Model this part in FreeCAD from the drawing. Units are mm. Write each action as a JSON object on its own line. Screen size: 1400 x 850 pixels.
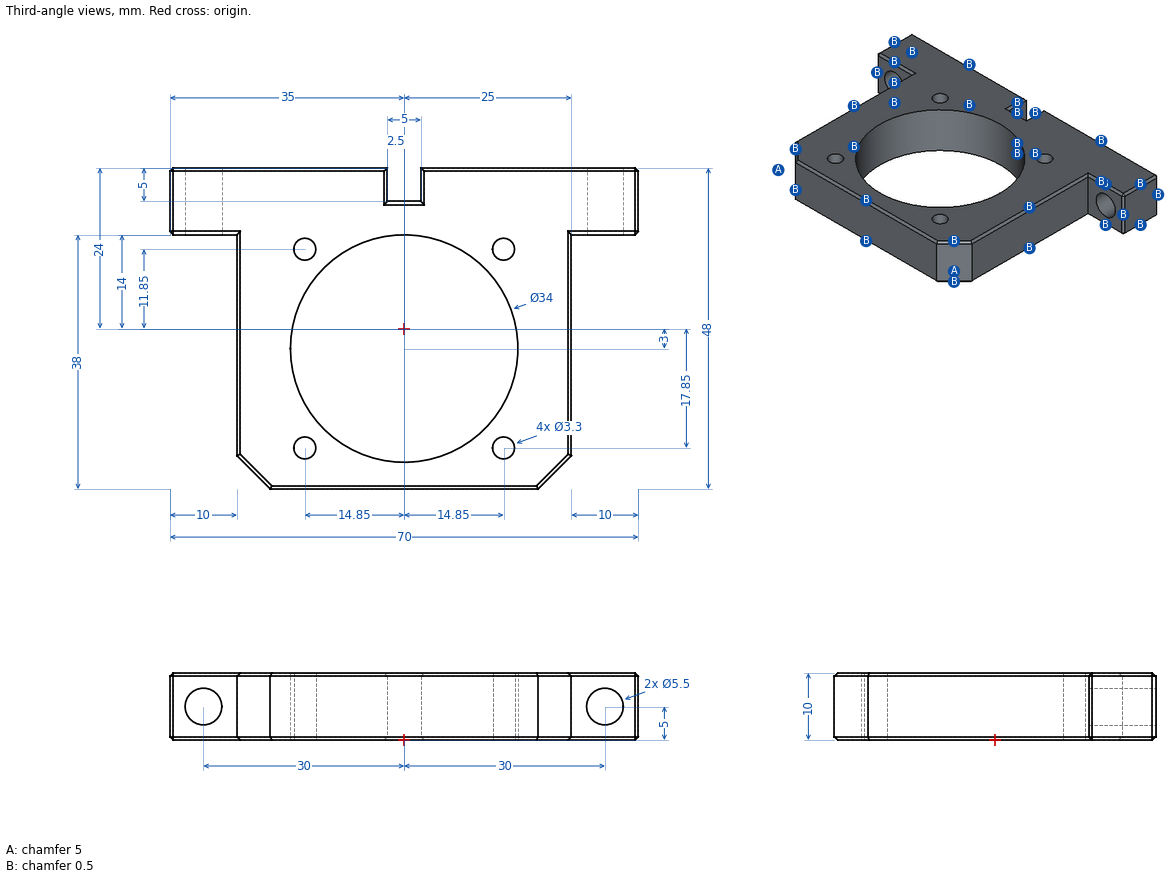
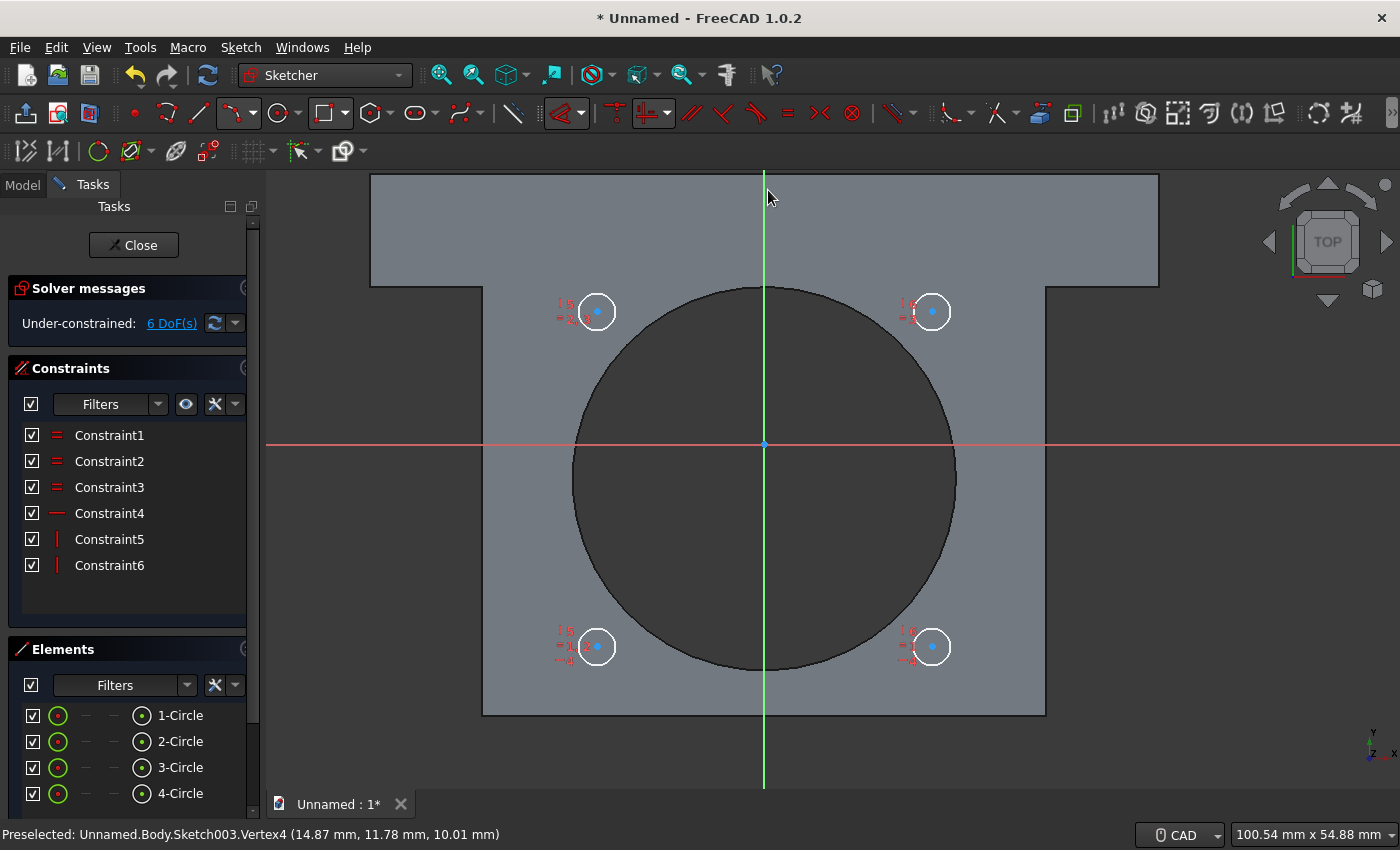
{"action": "left_click", "coordinate": [597, 312]}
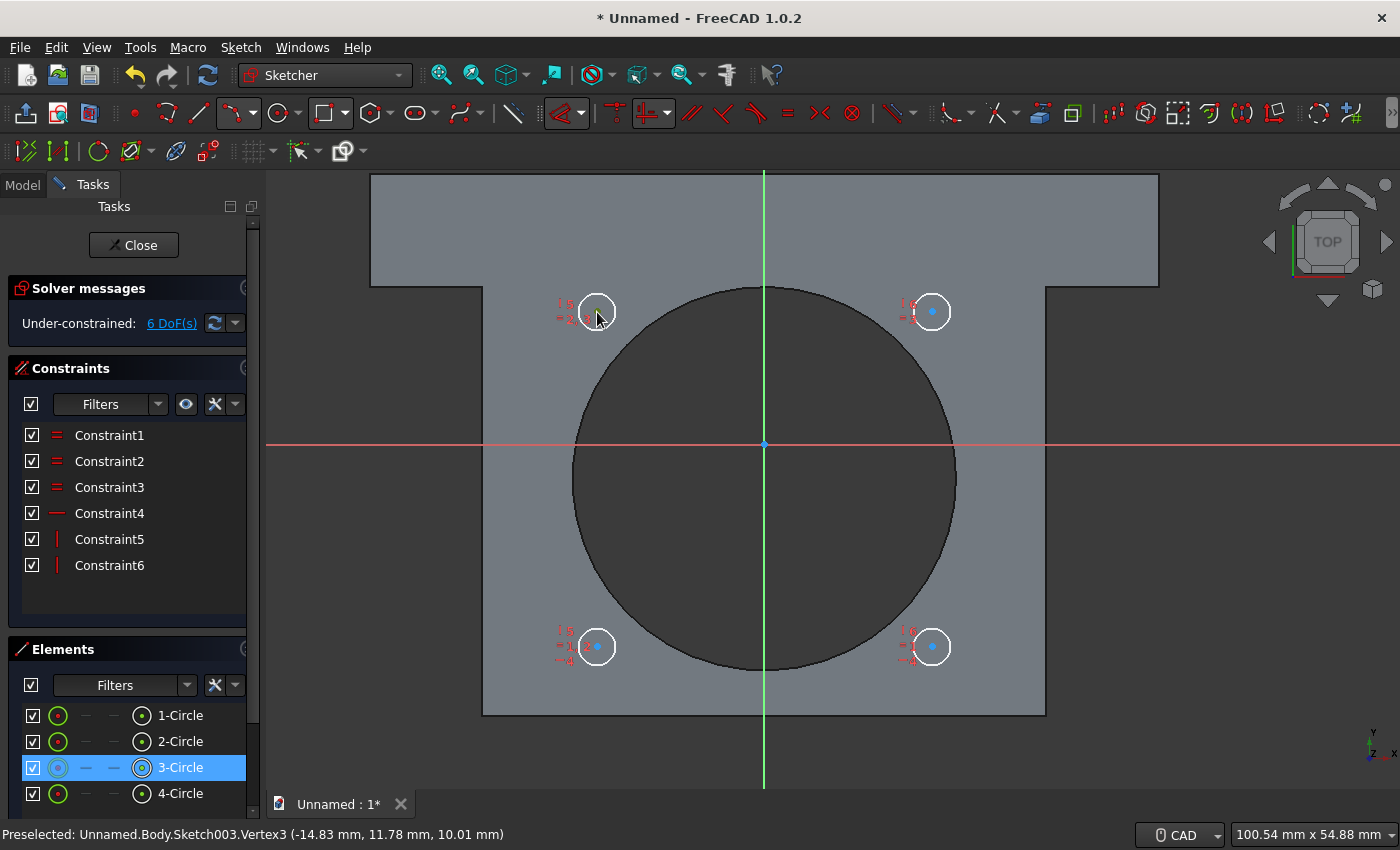
{"action": "left_click", "coordinate": [932, 312]}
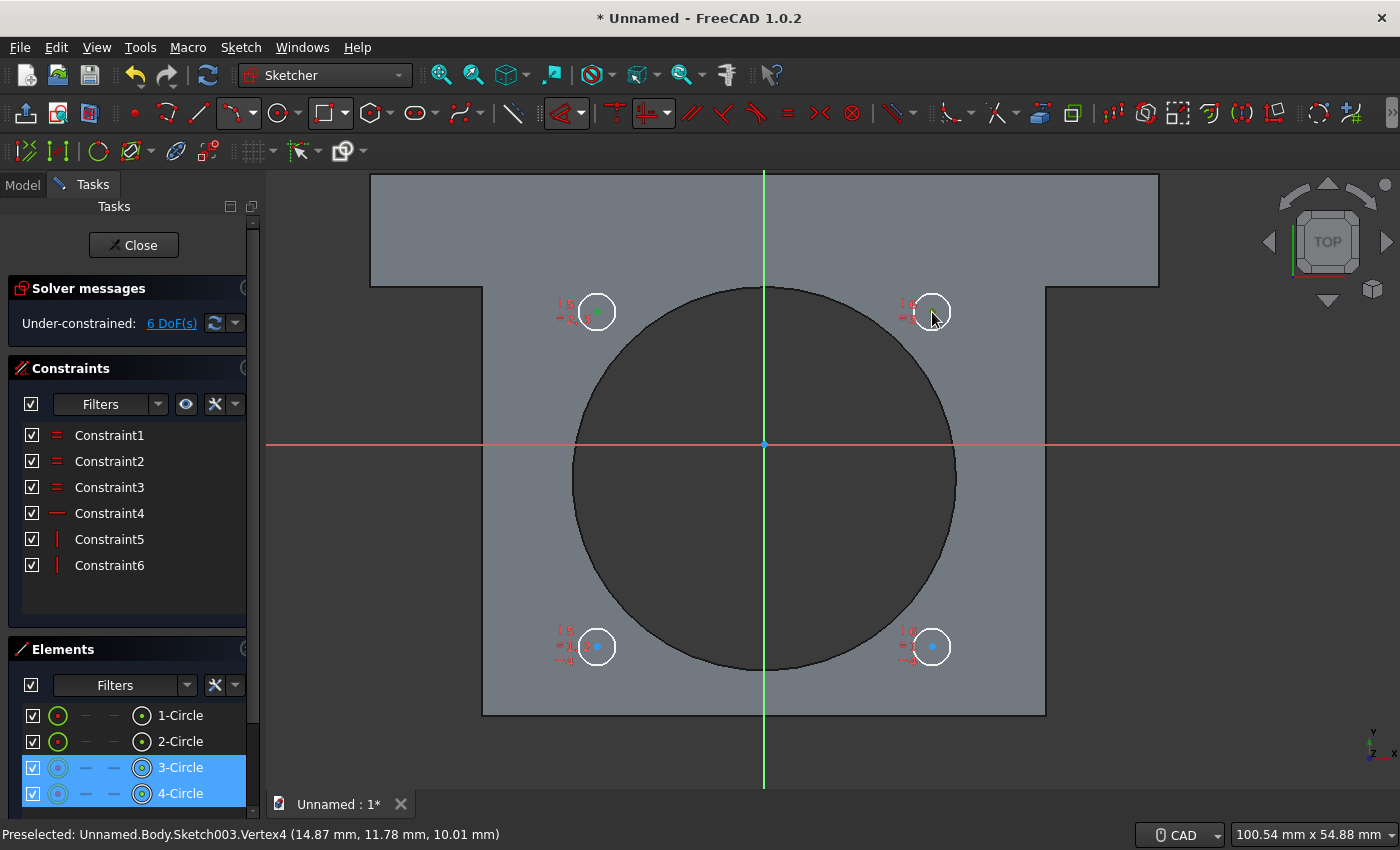
{"action": "left_click", "coordinate": [670, 114]}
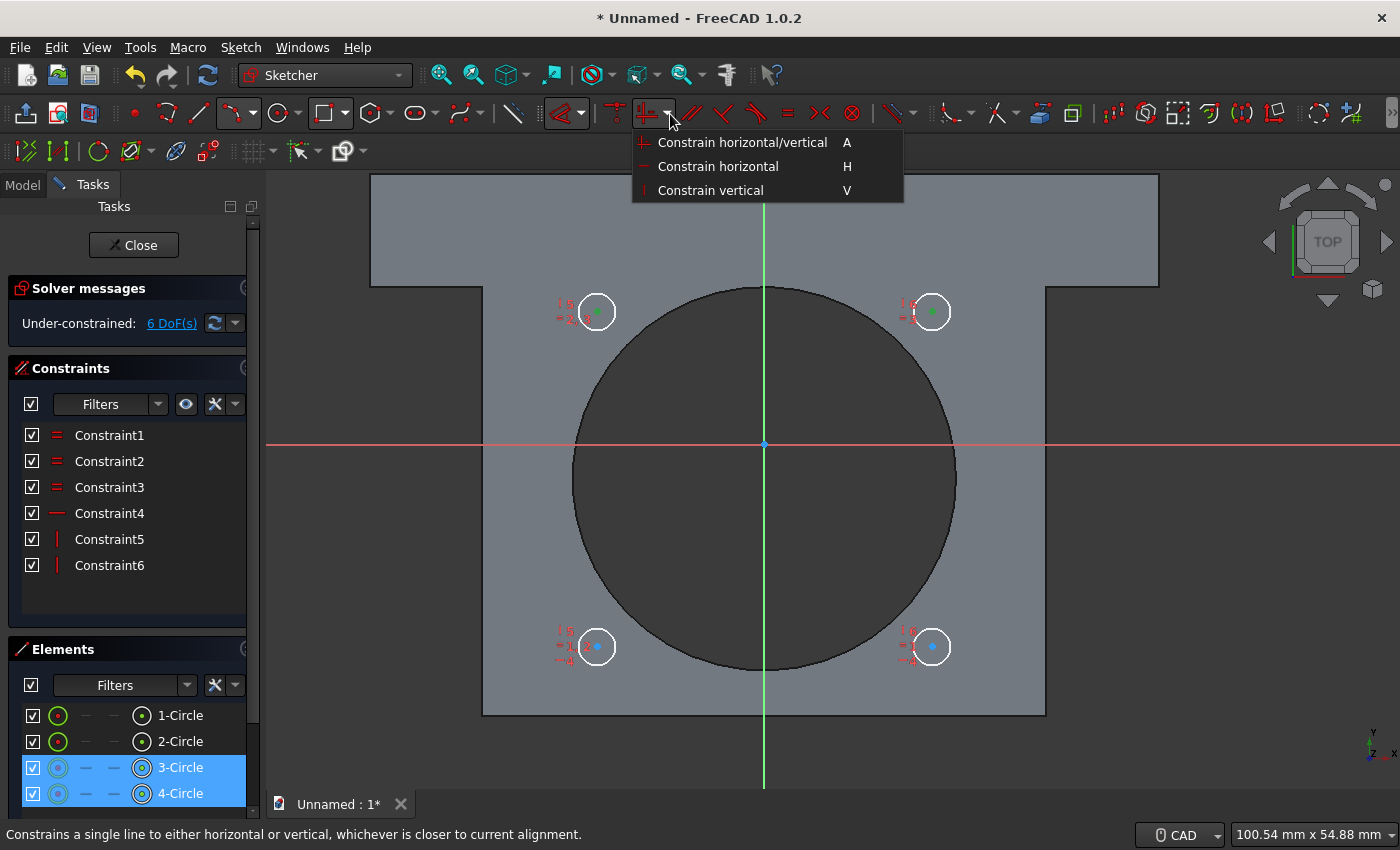
{"action": "left_click", "coordinate": [768, 166]}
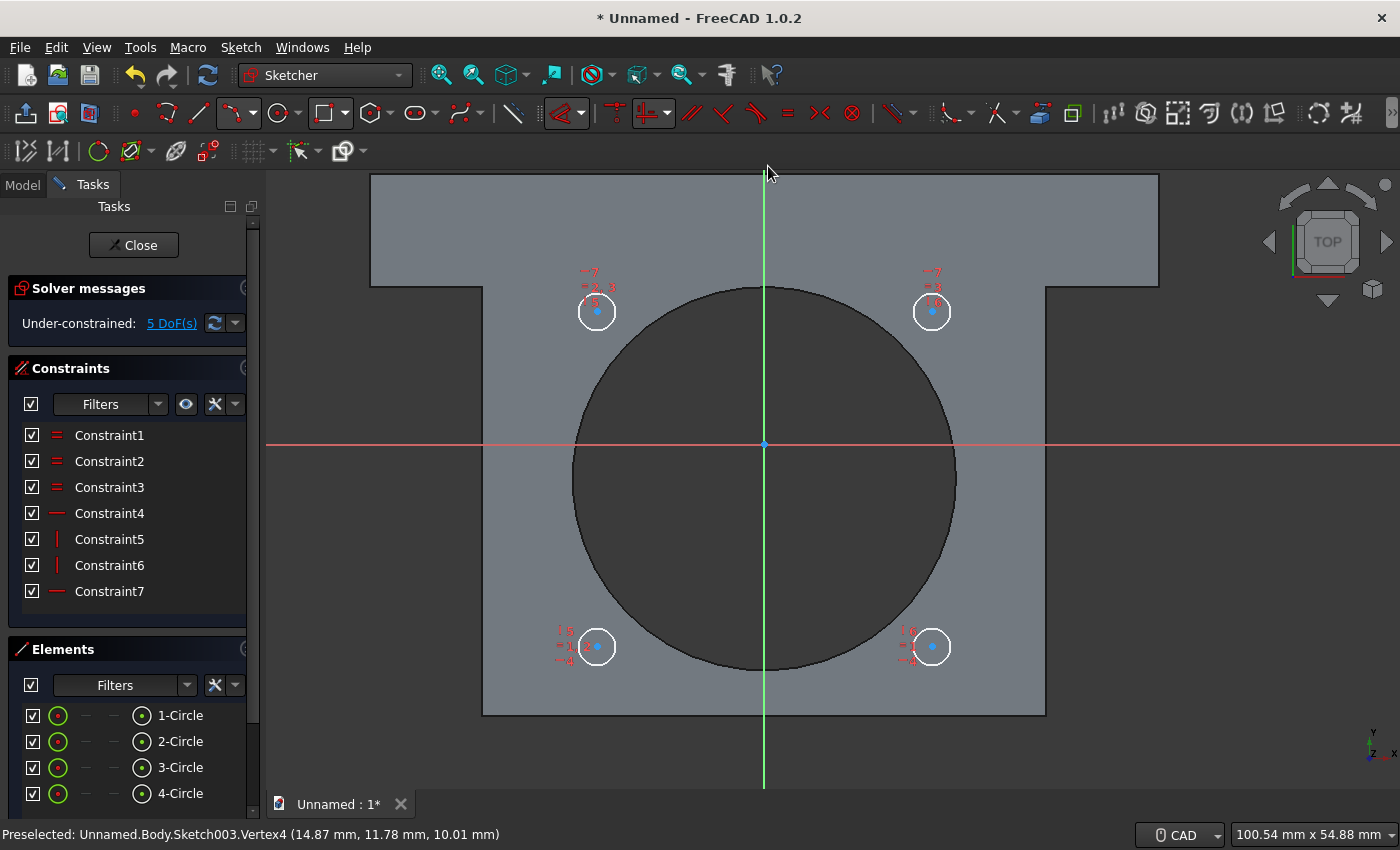
{"action": "left_click", "coordinate": [945, 634]}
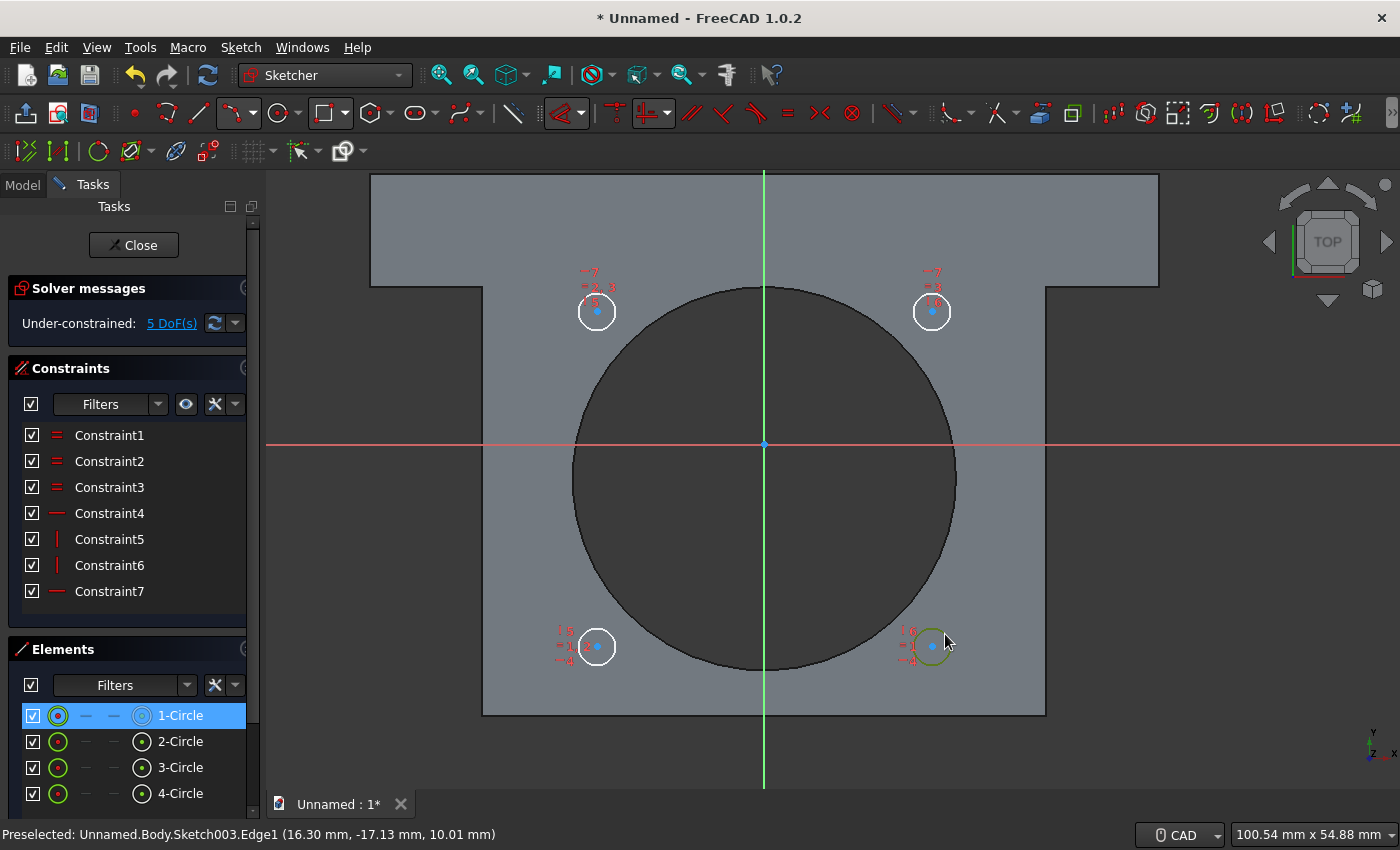
{"action": "key", "text": "k o"}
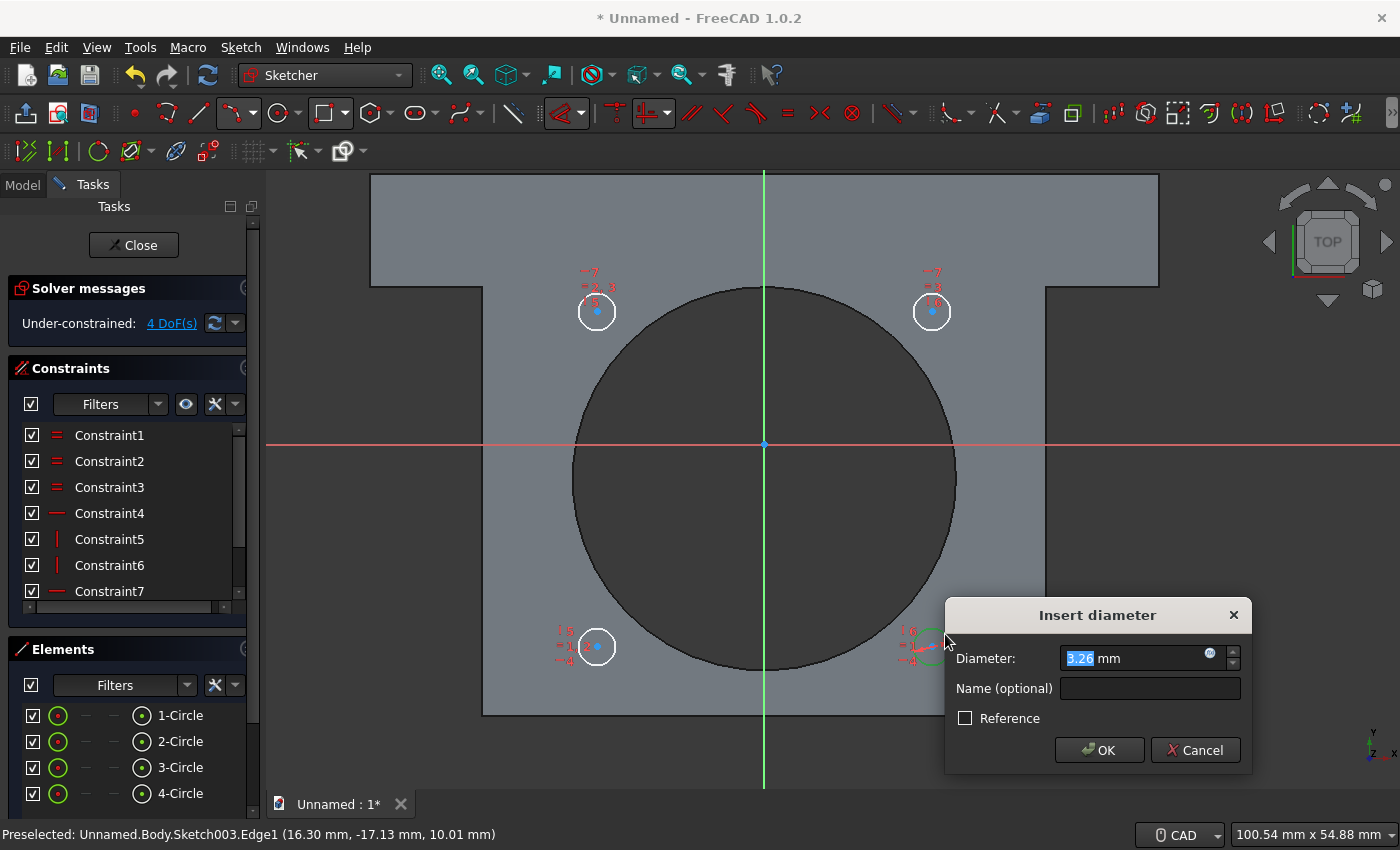
{"action": "type", "text": "3.3"}
{"action": "key", "text": "Return"}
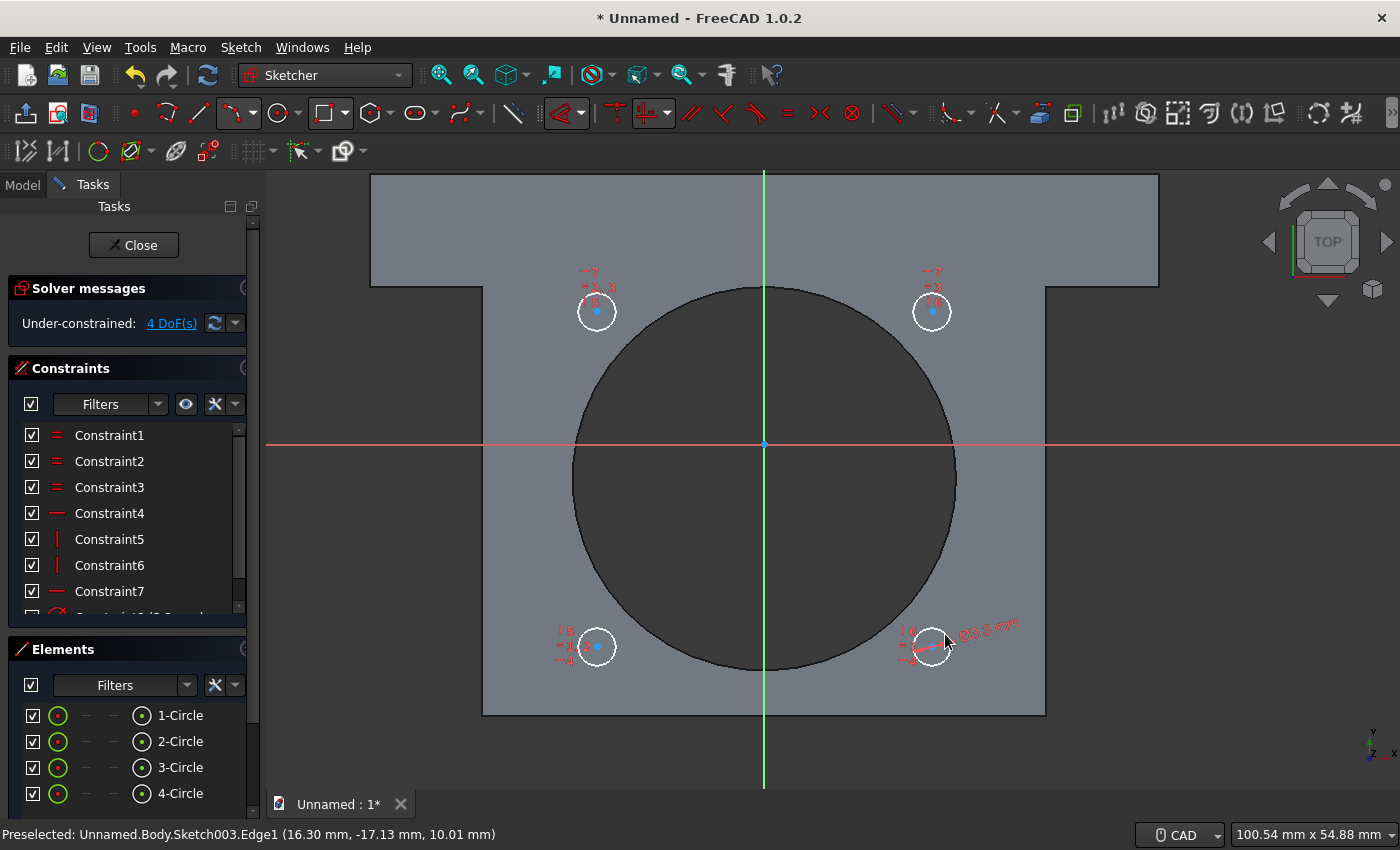
{"action": "left_click", "coordinate": [932, 647]}